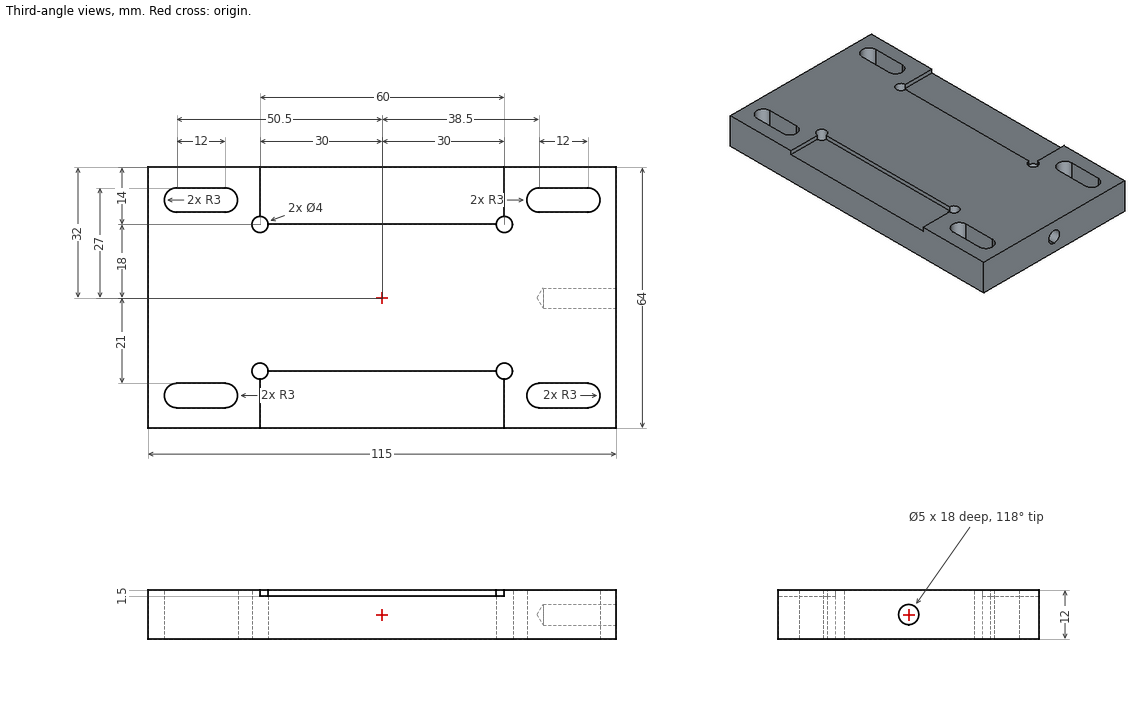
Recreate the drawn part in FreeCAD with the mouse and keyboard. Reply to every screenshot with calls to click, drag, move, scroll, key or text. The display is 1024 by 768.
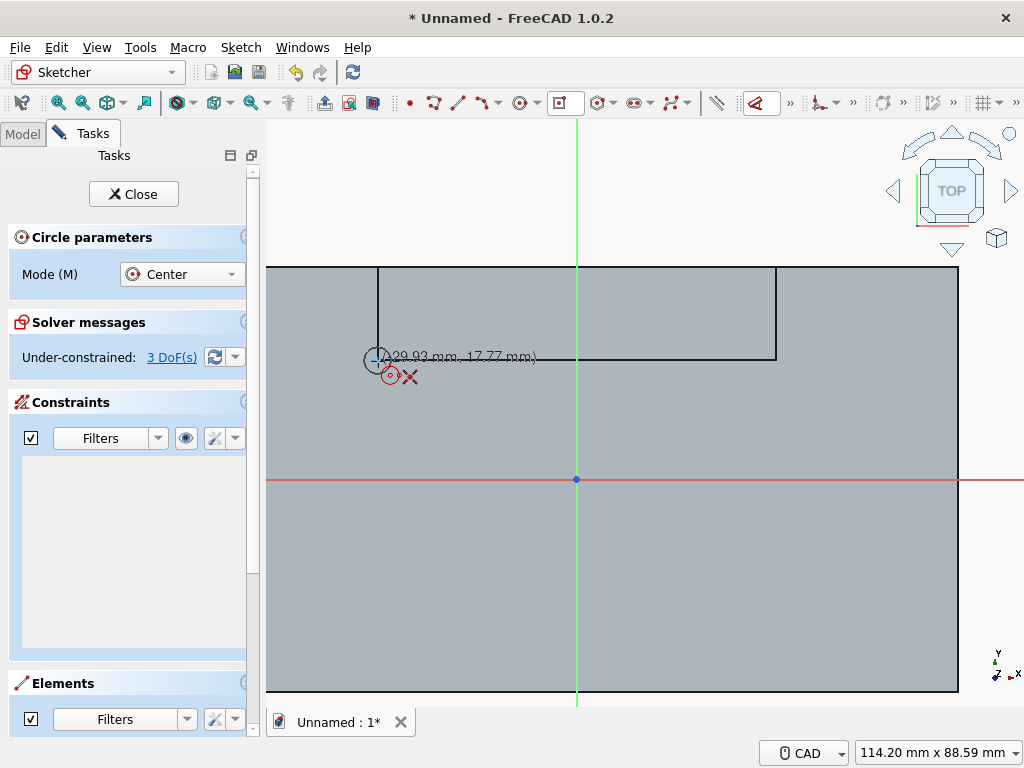
scroll(776, 360, up, 3)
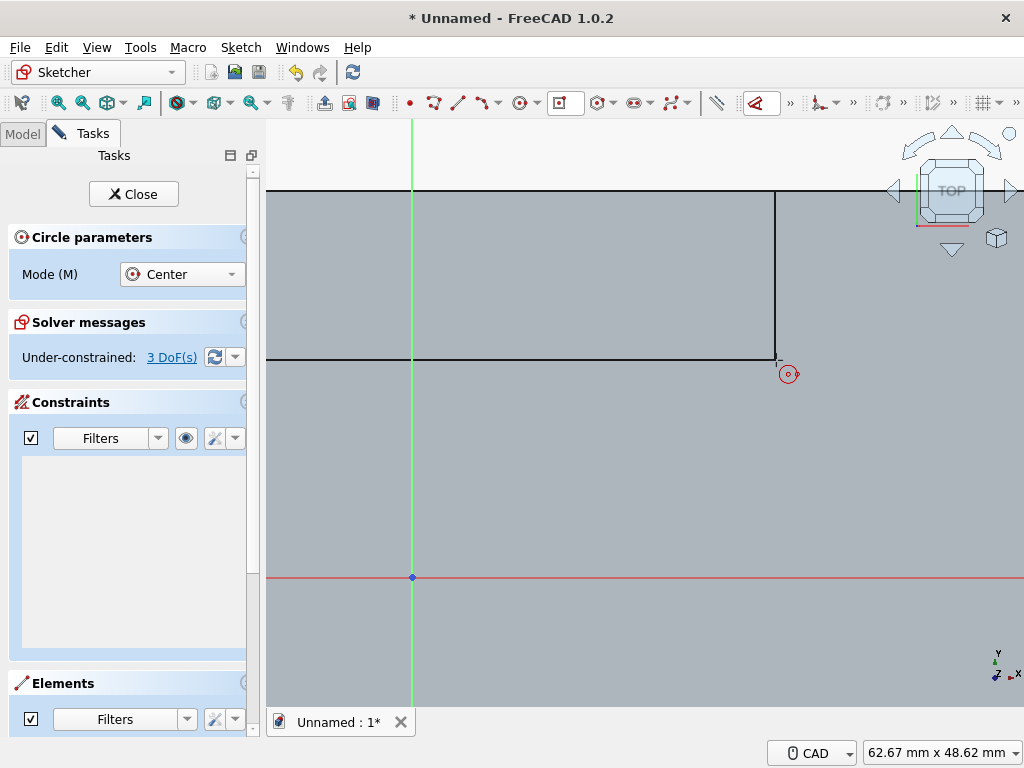
click(775, 360)
click(792, 343)
key(Escape)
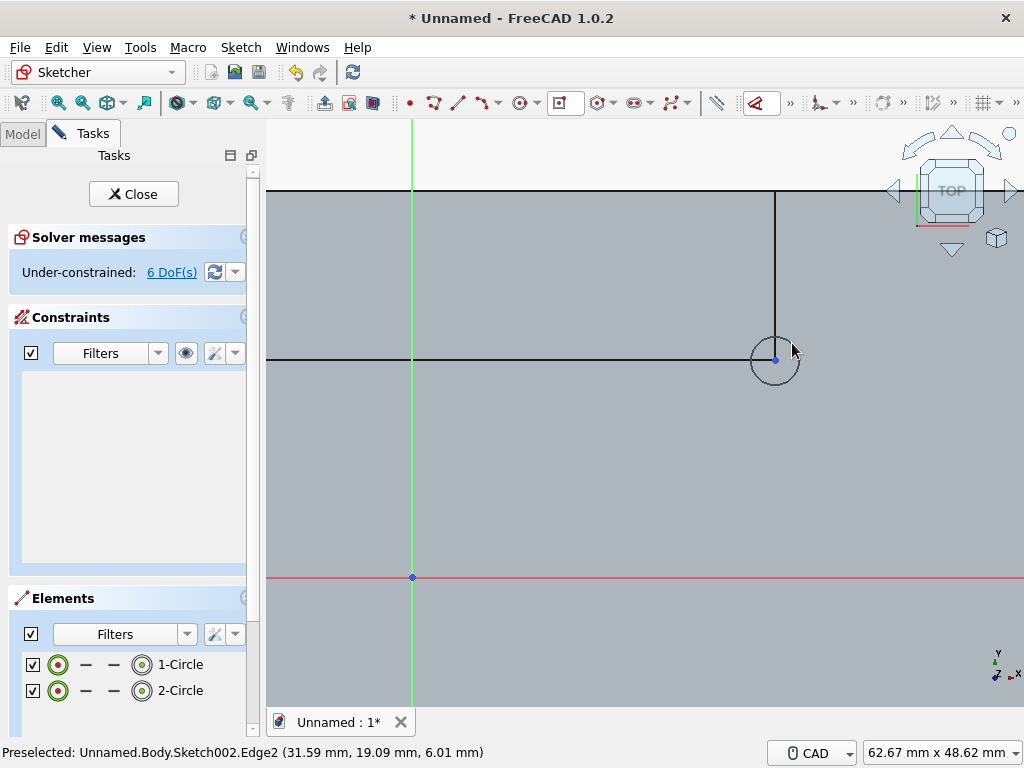
scroll(776, 360, down, 3)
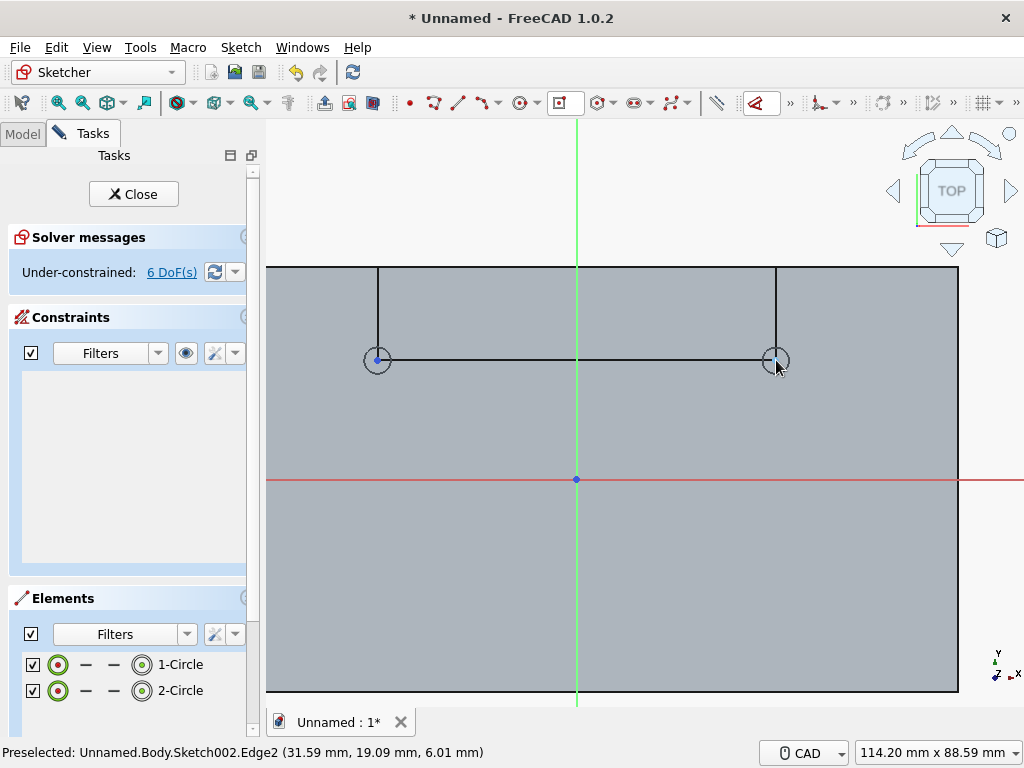
click(387, 351)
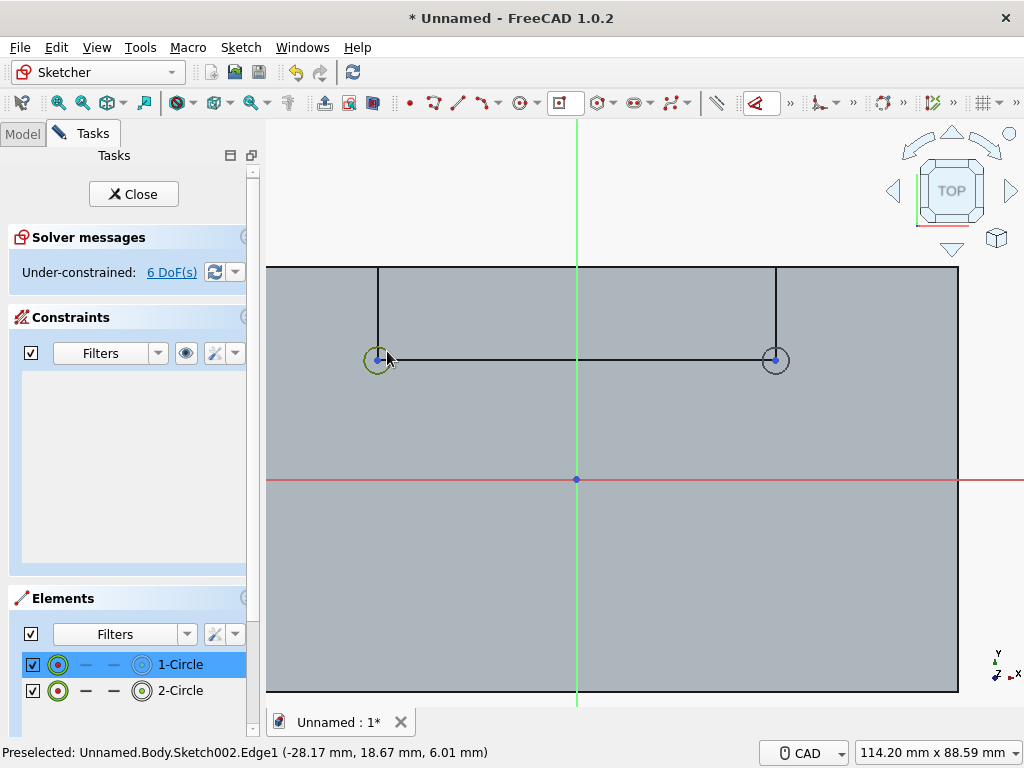
click(785, 351)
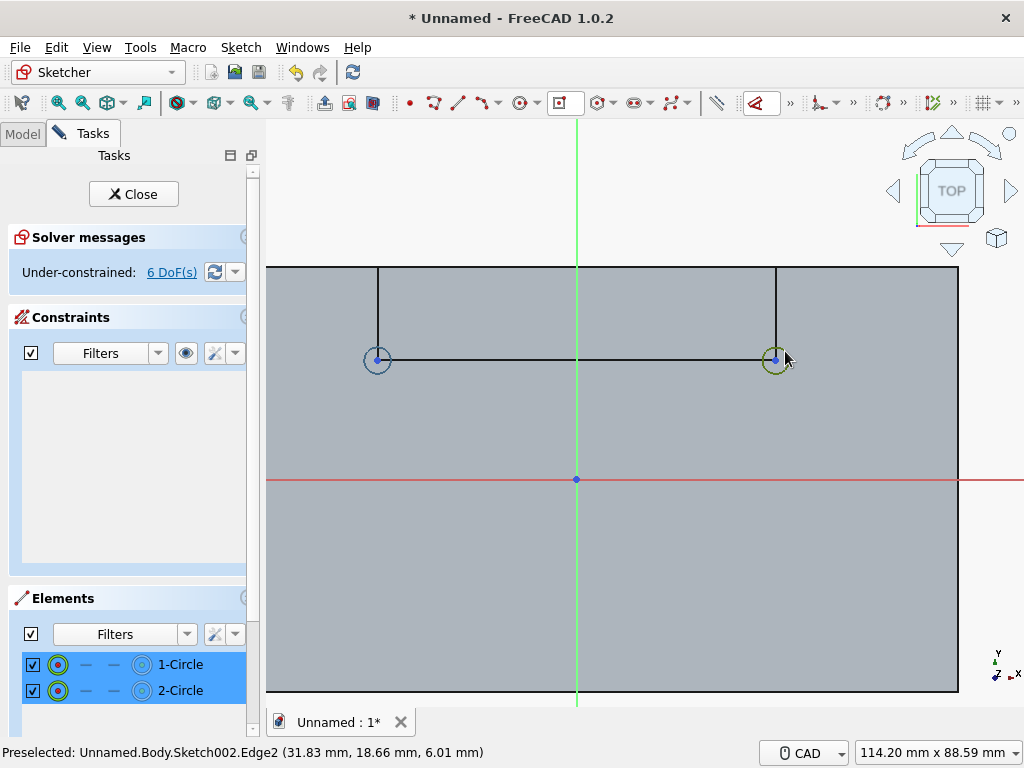
key(e)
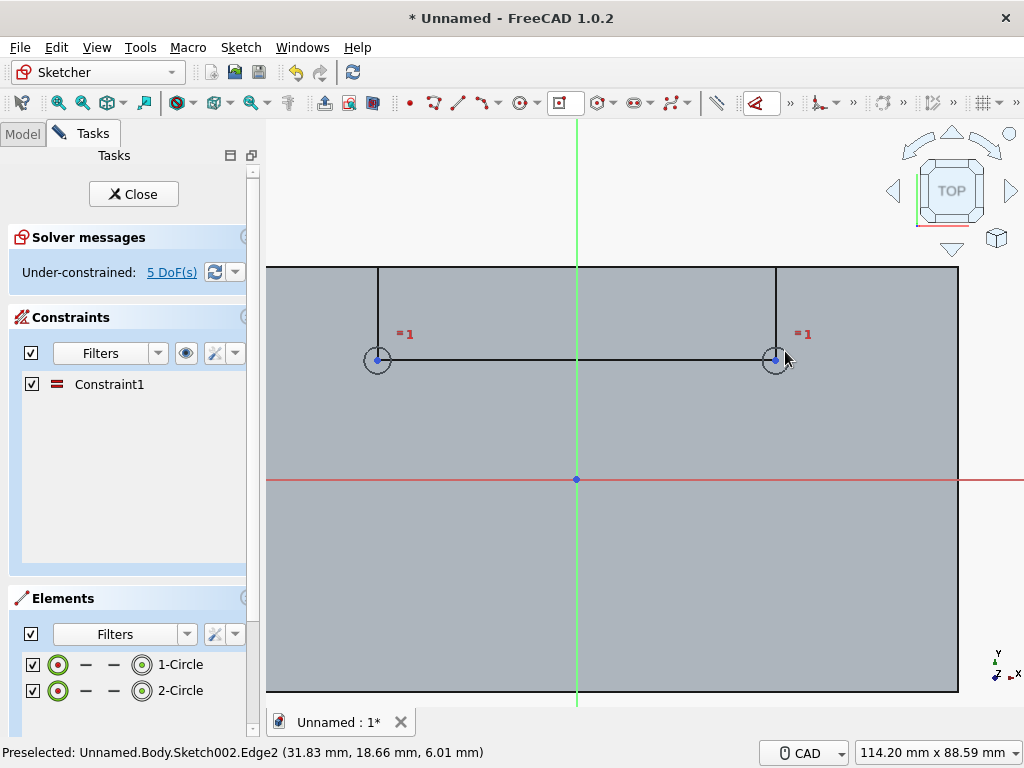
scroll(387, 351, up, 3)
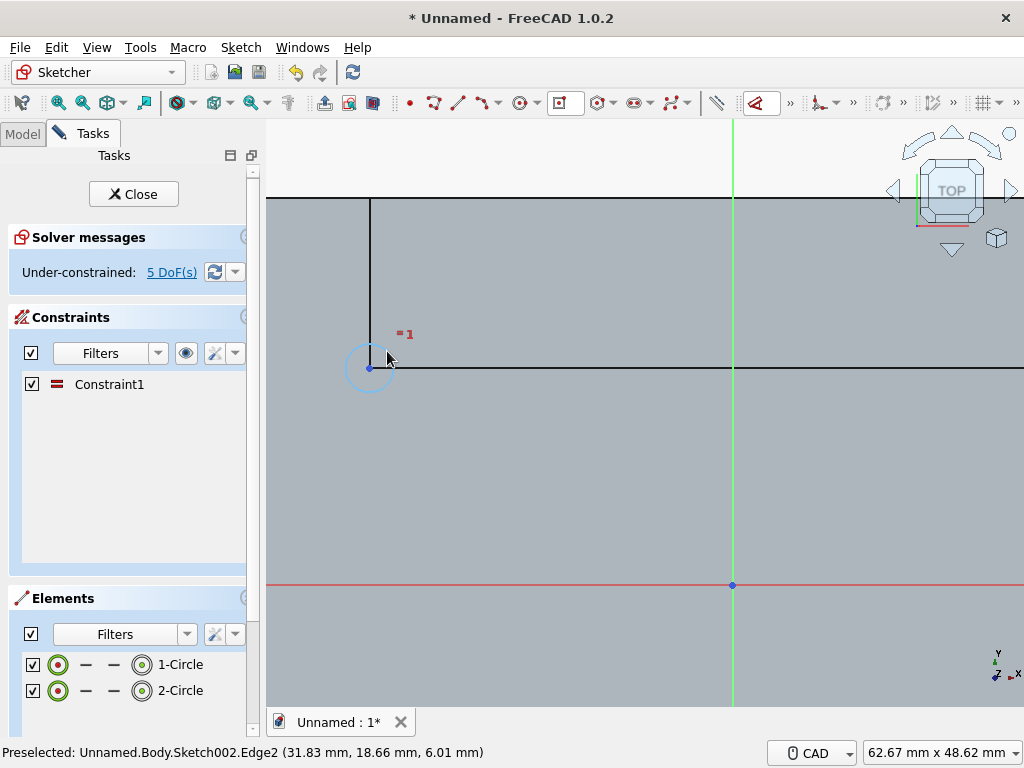
click(387, 351)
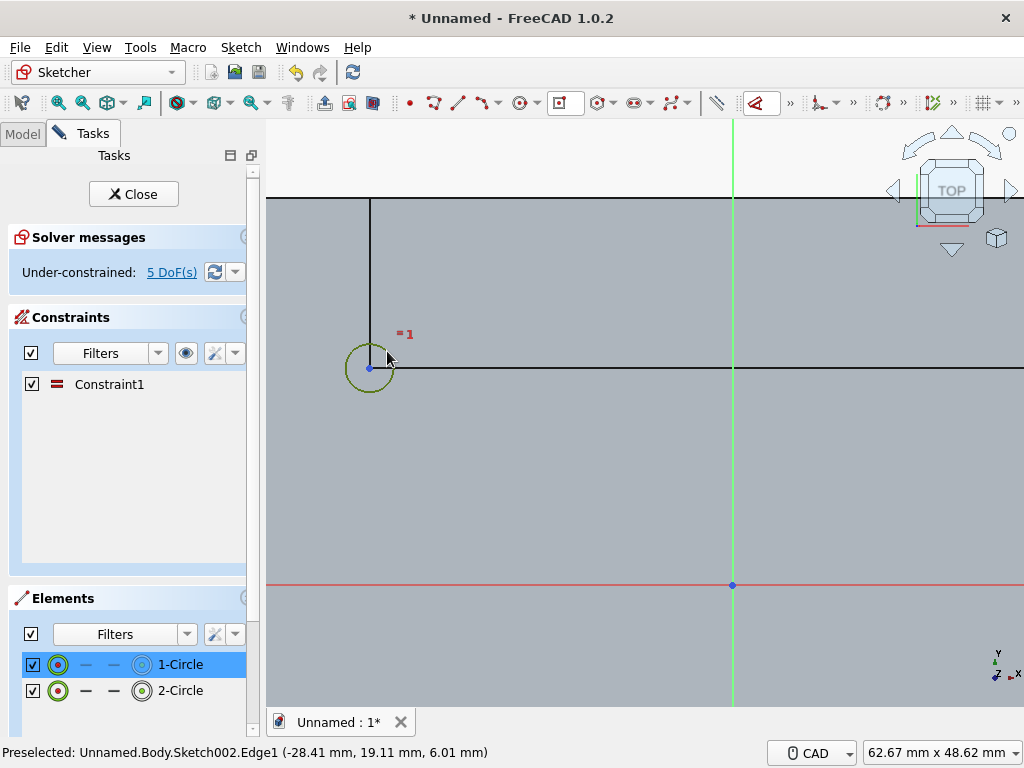
click(774, 104)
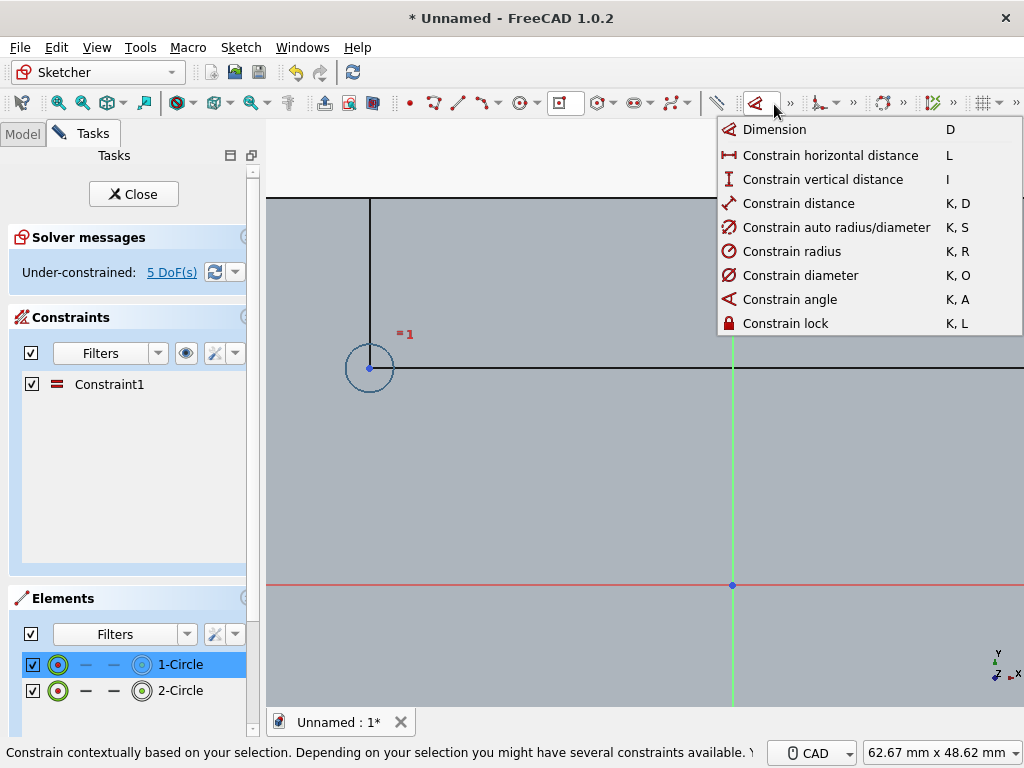
click(870, 275)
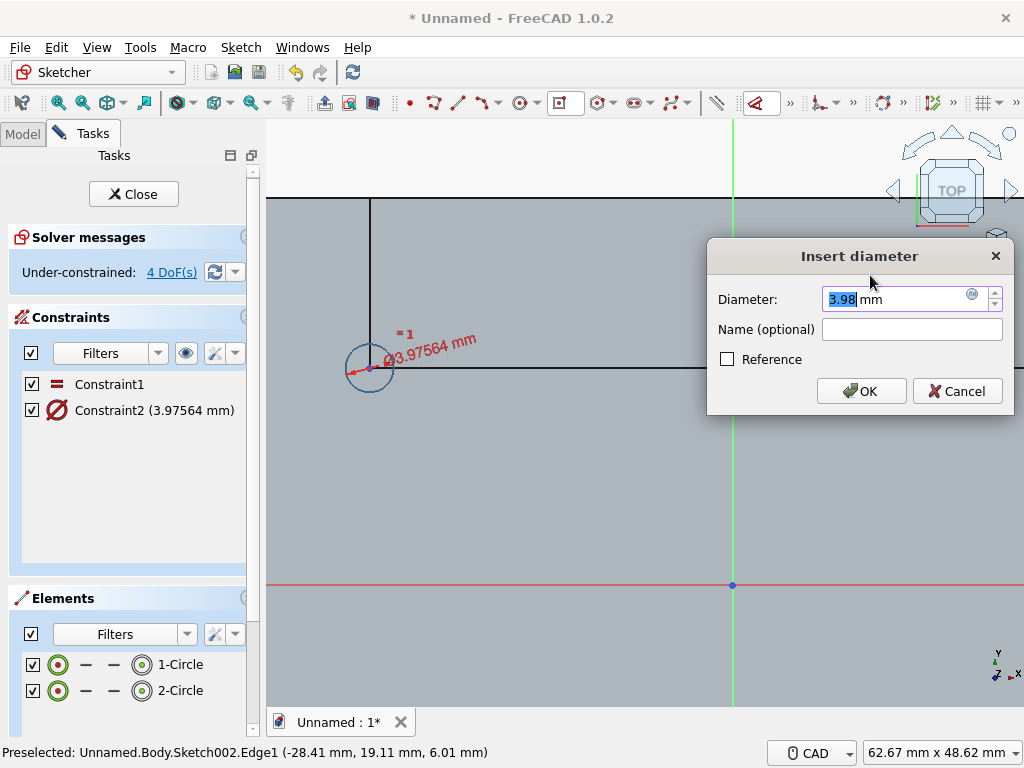
text(4)
key(Return)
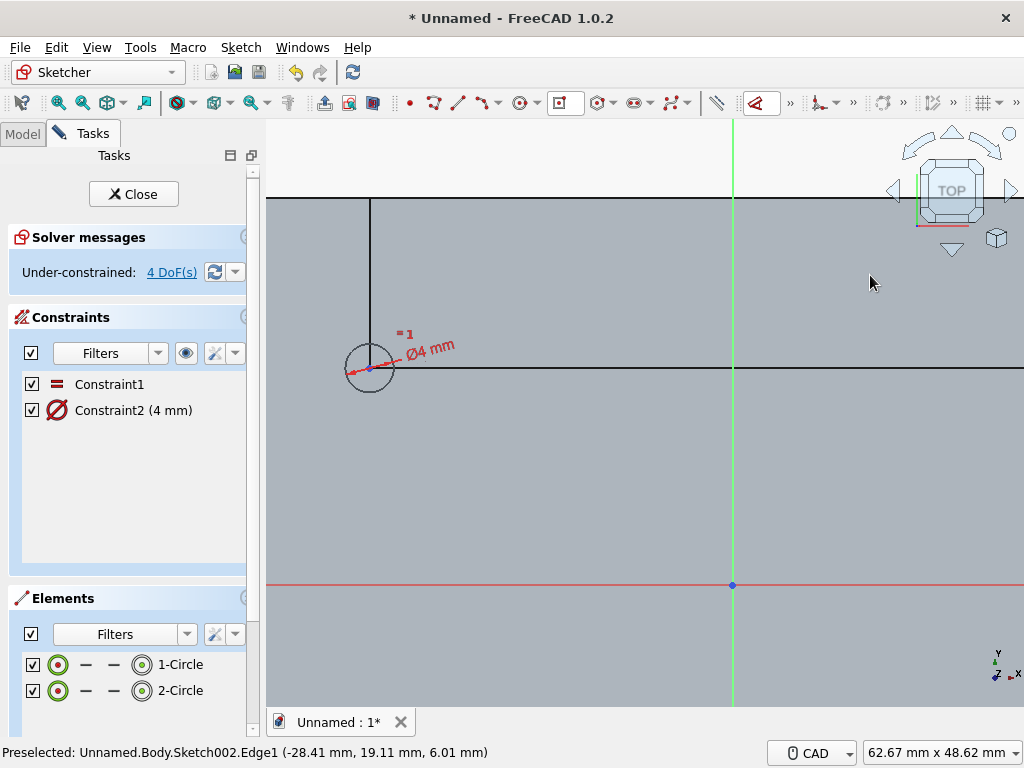
click(370, 368)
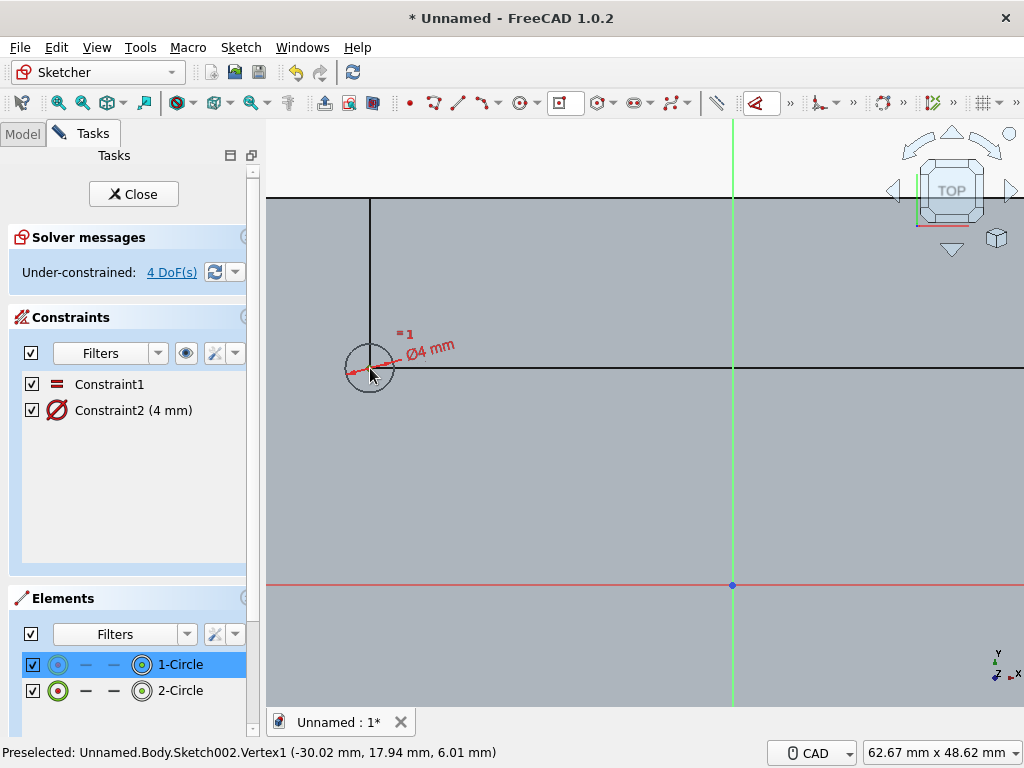
key(l)